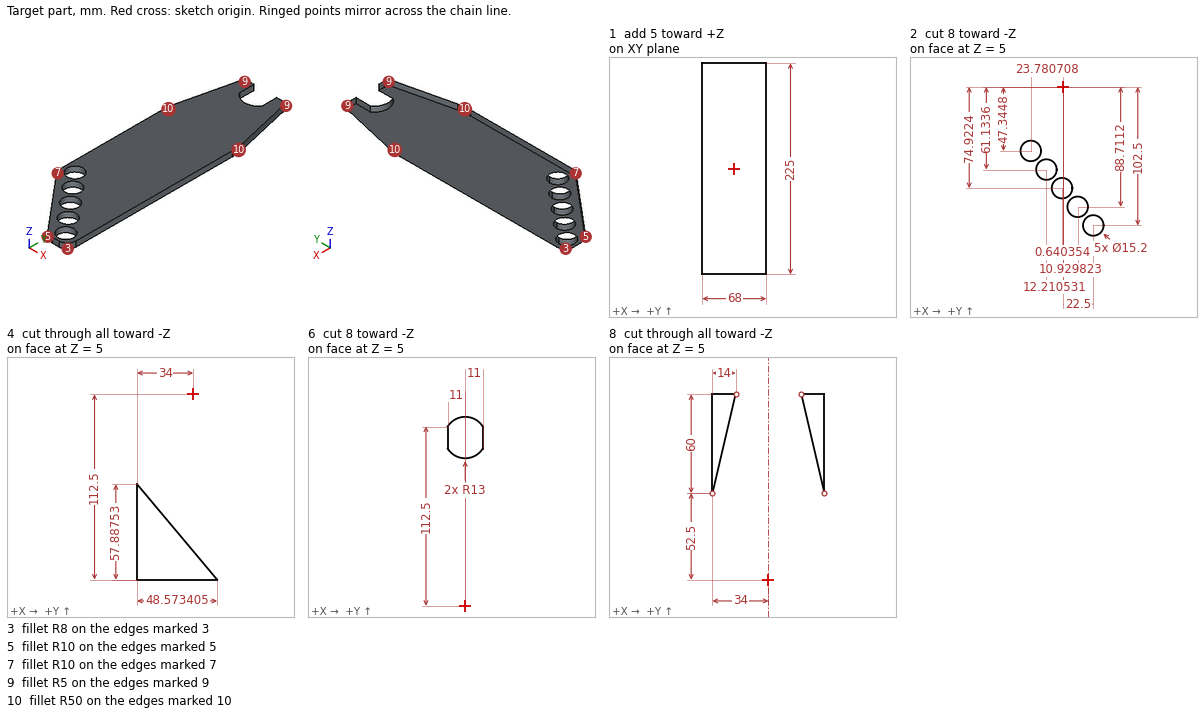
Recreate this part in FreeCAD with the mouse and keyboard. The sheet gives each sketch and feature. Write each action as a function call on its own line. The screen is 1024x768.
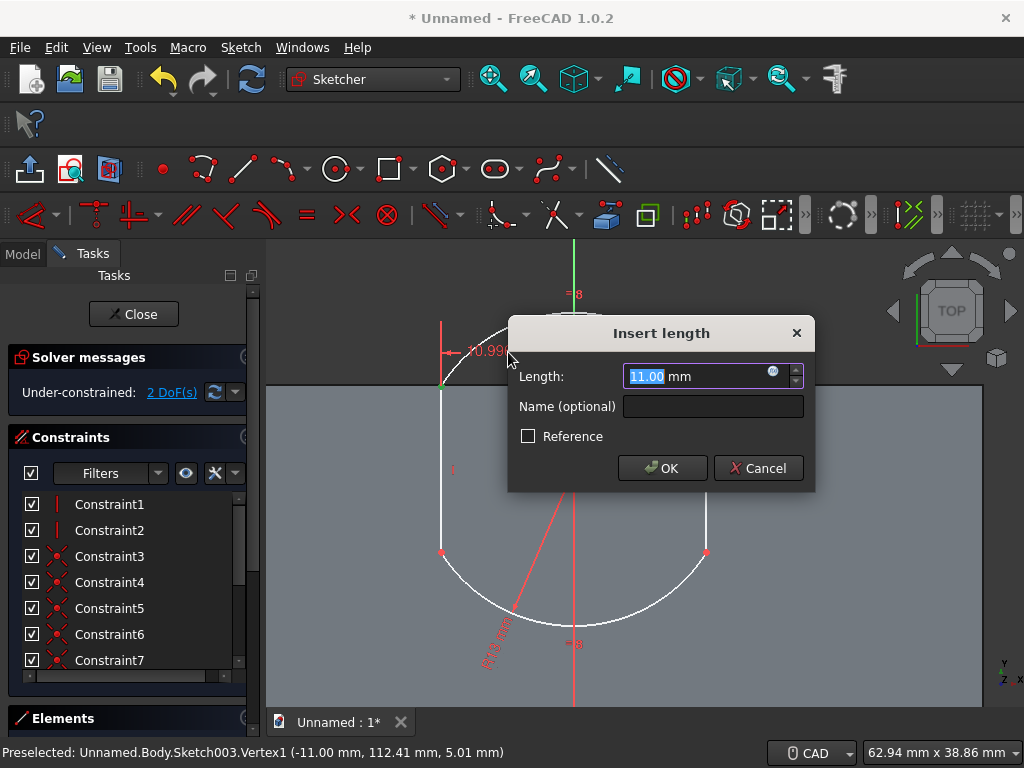
text(11)
key(Return)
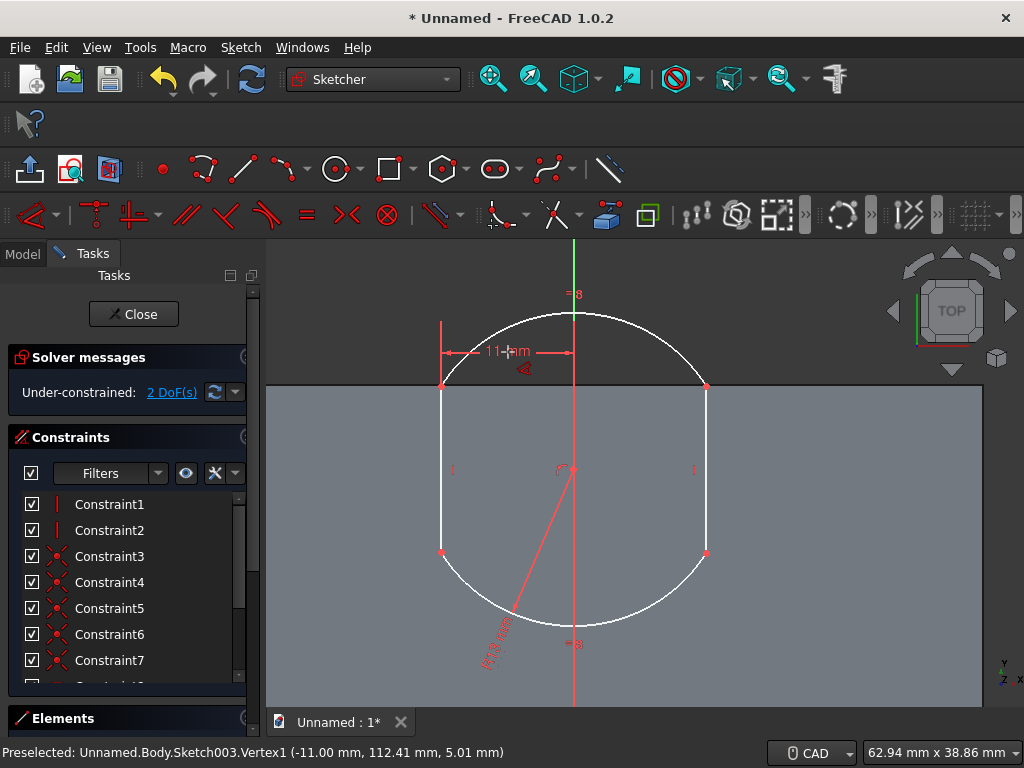
click(706, 553)
click(640, 519)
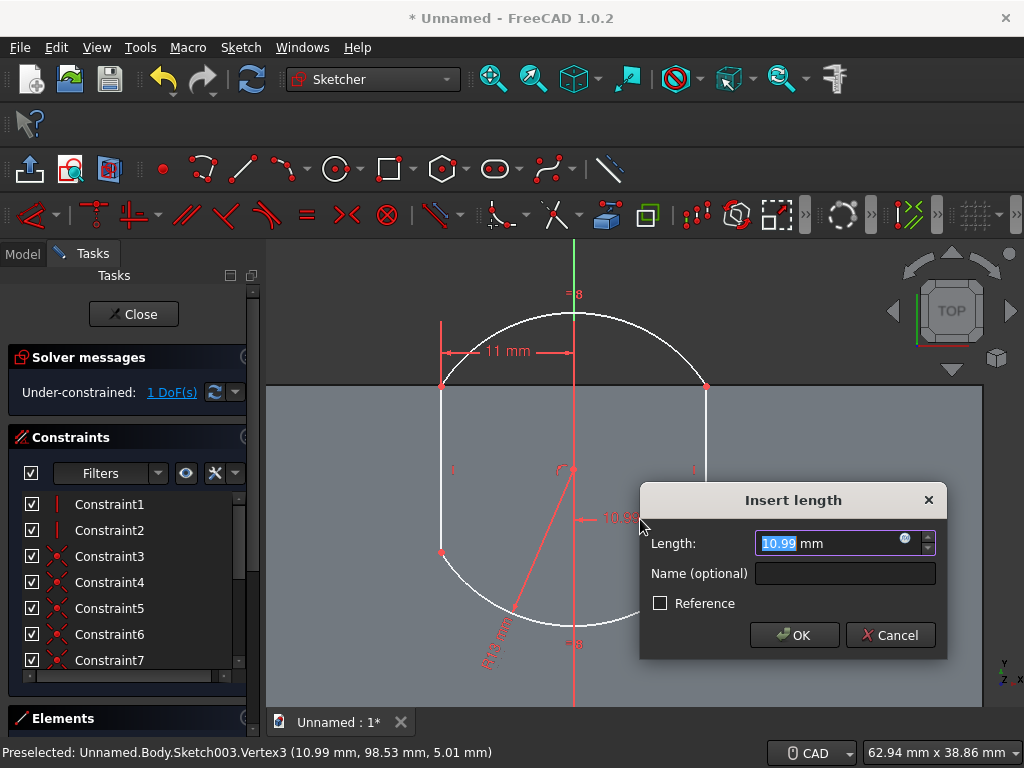
text(11)
key(Return)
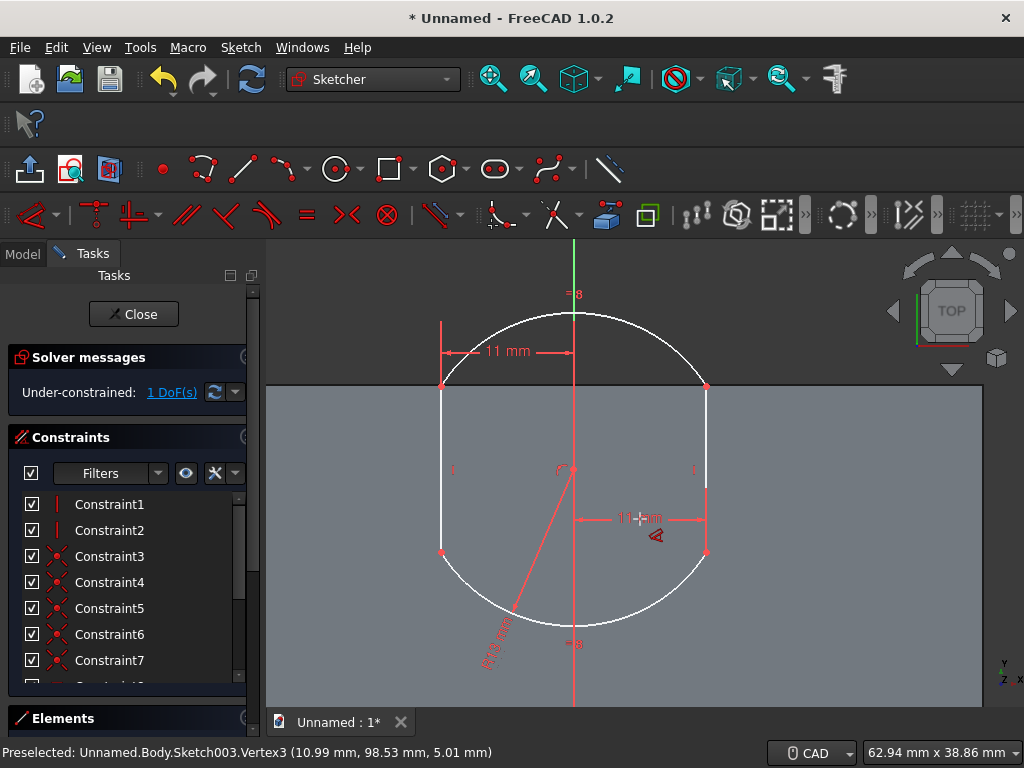
click(441, 386)
click(407, 533)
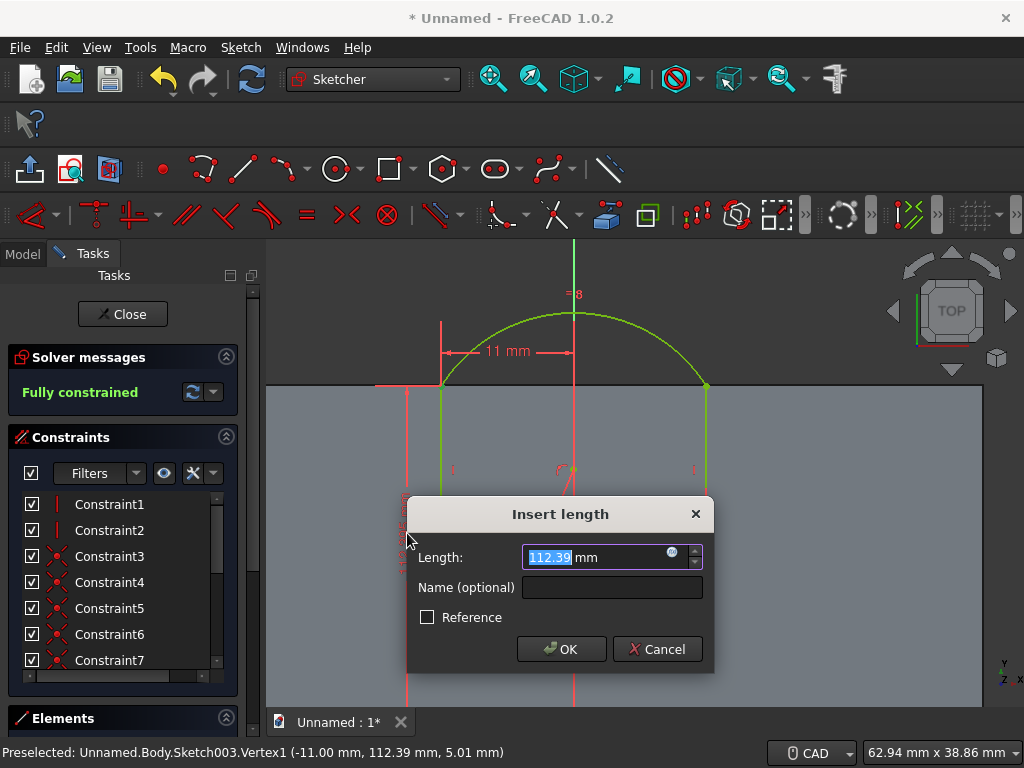
text(112.5)
key(Return)
key(Escape)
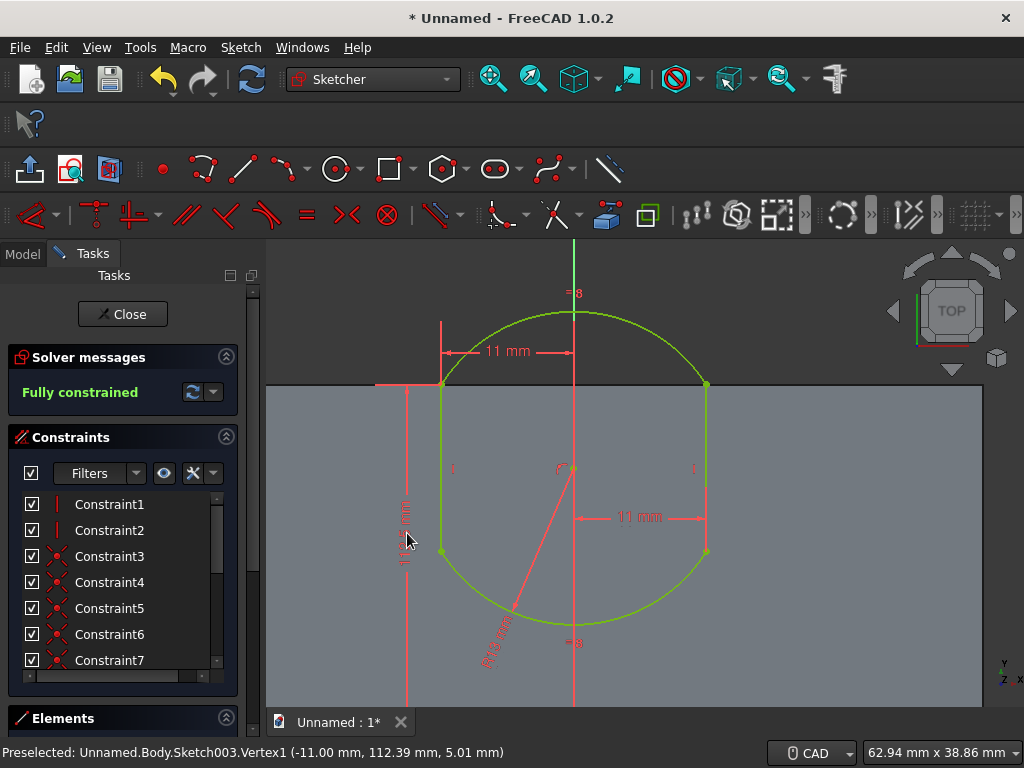
click(123, 314)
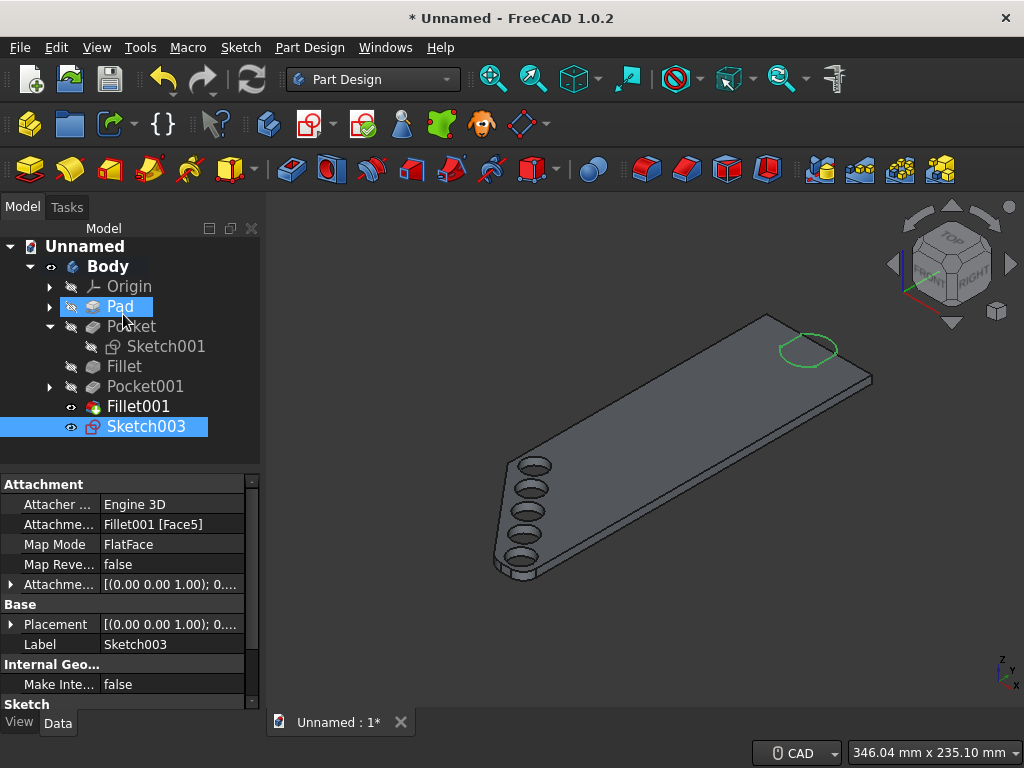
click(292, 170)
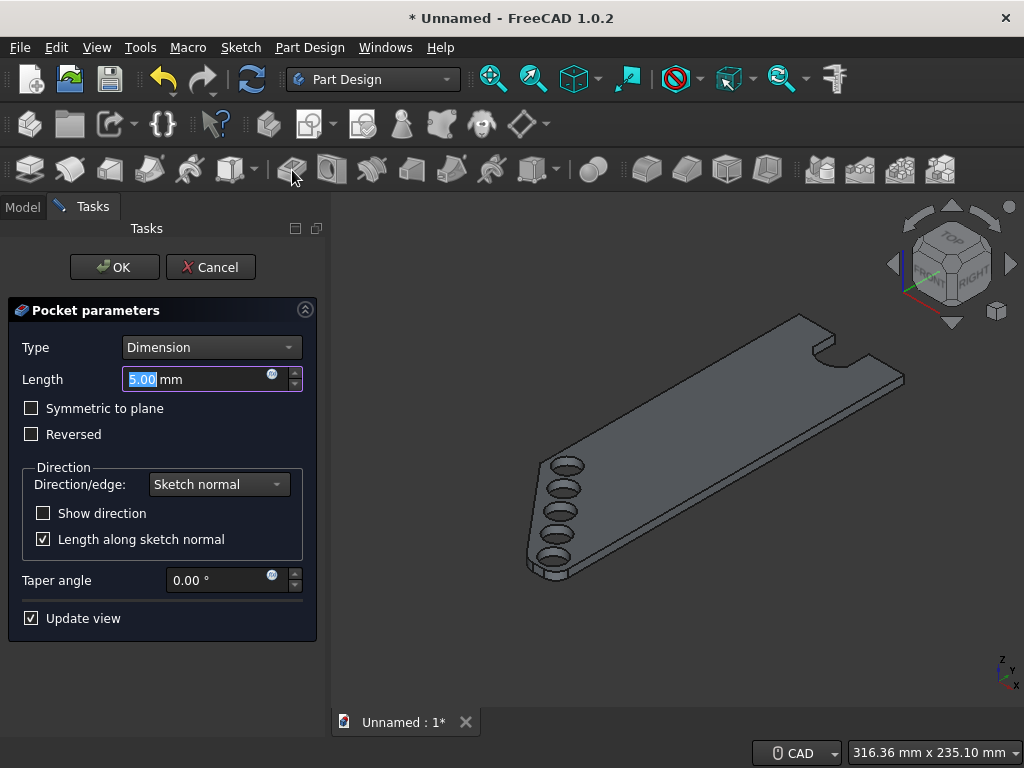
text(8)
key(Tab)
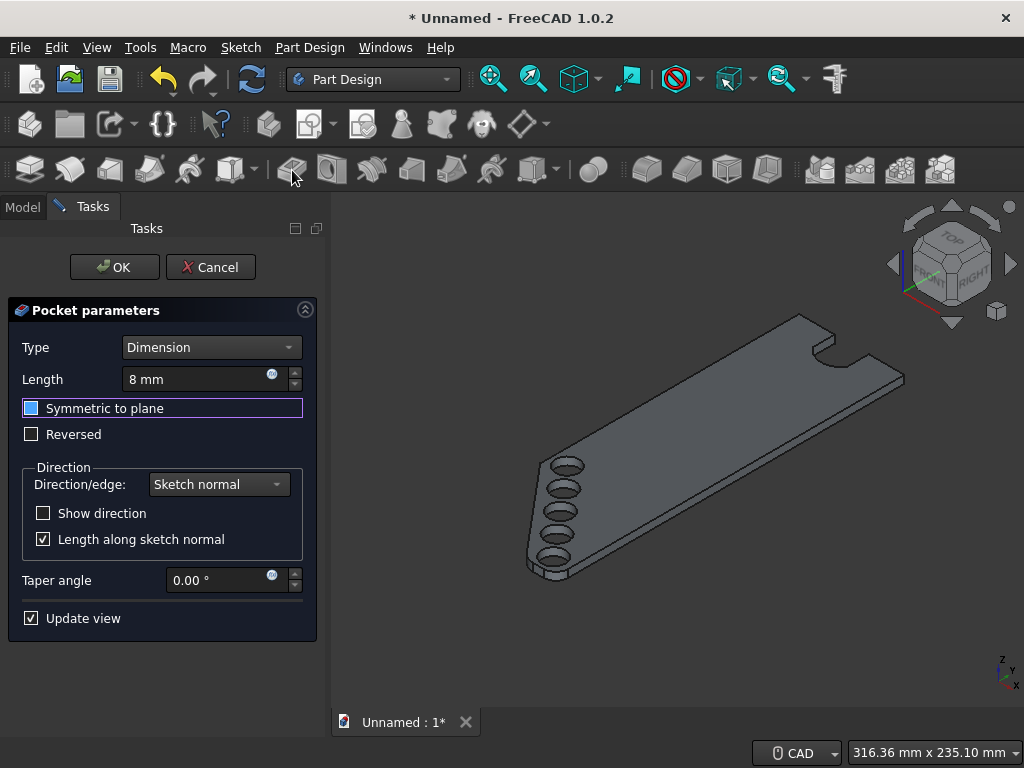
click(115, 267)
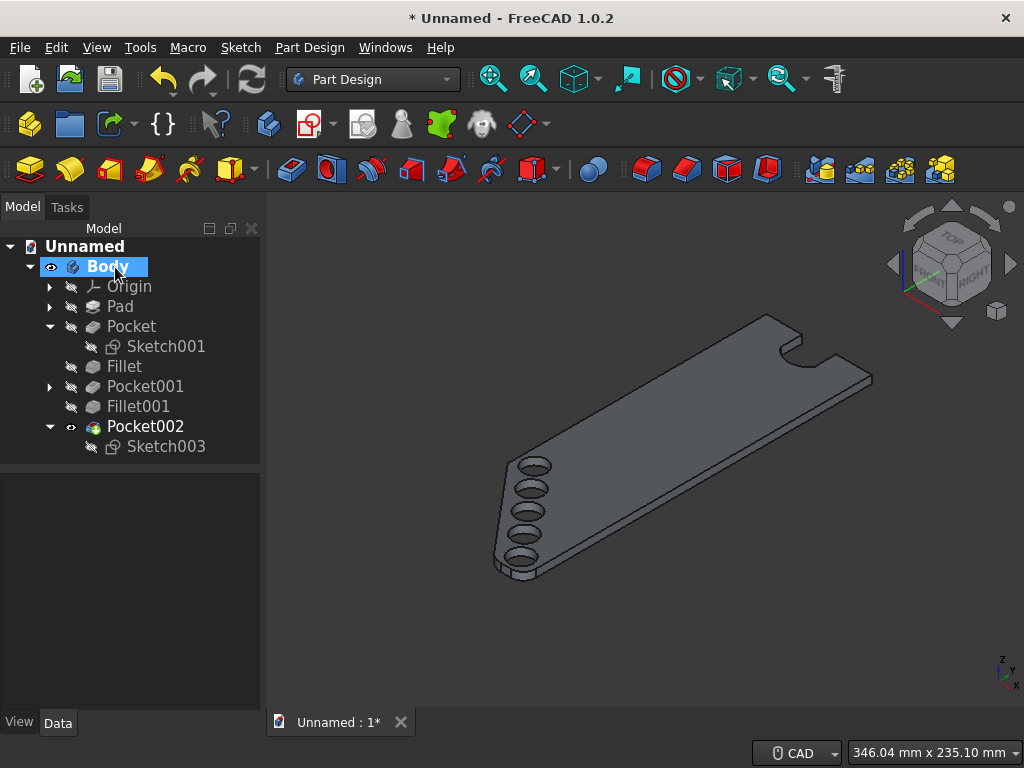
scroll(508, 467, up, 7)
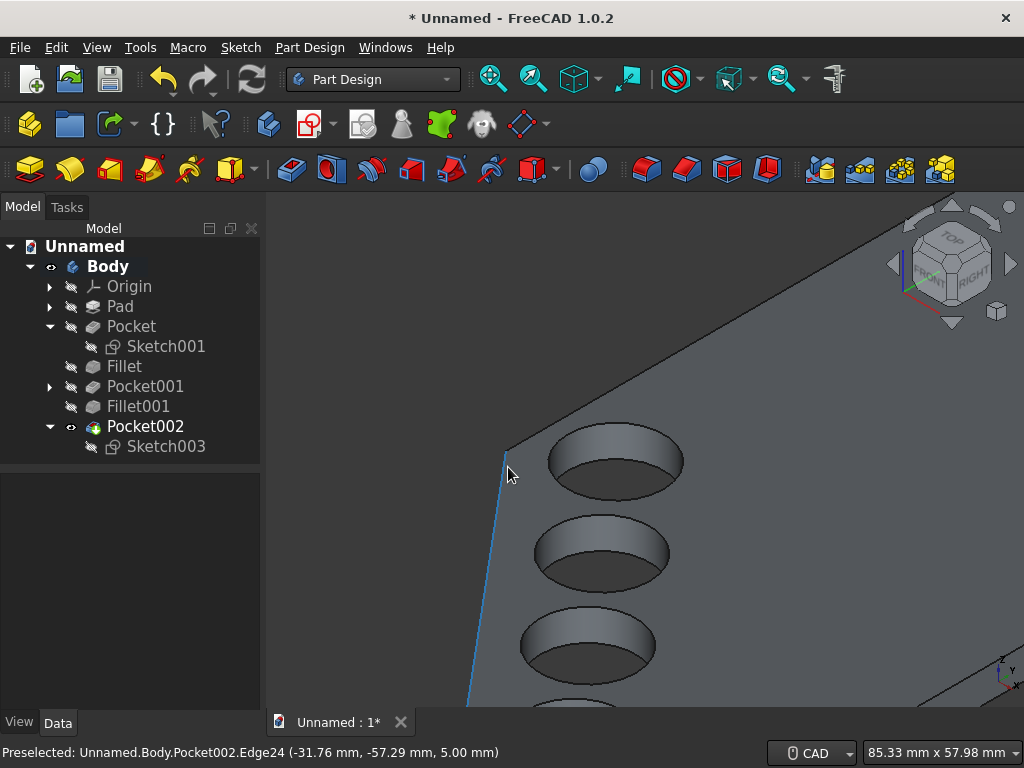
key(v)
key(f)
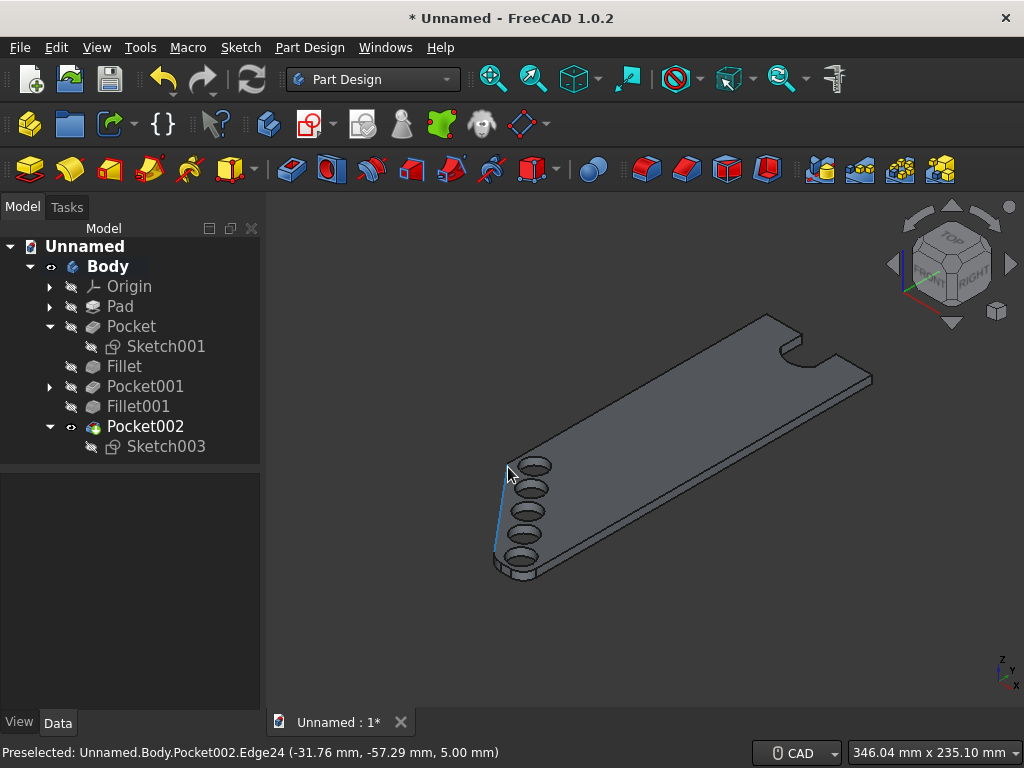
key(2)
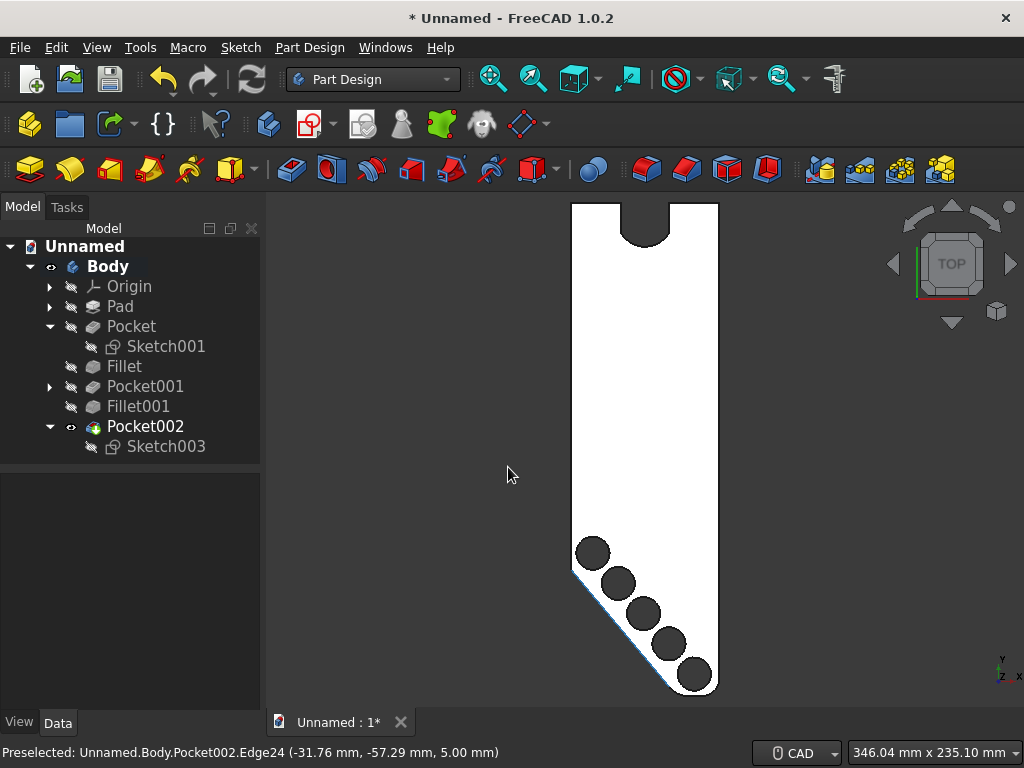
scroll(571, 568, up, 7)